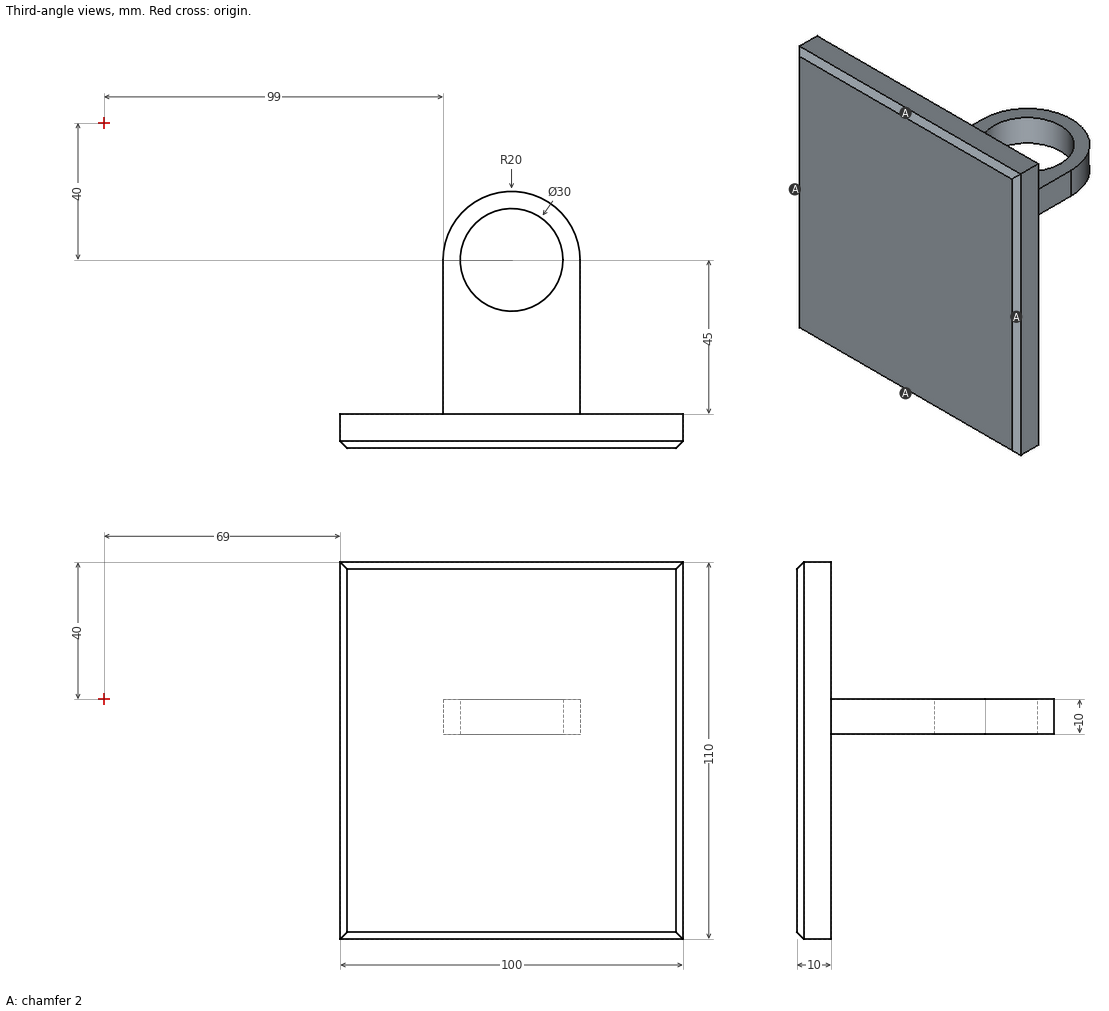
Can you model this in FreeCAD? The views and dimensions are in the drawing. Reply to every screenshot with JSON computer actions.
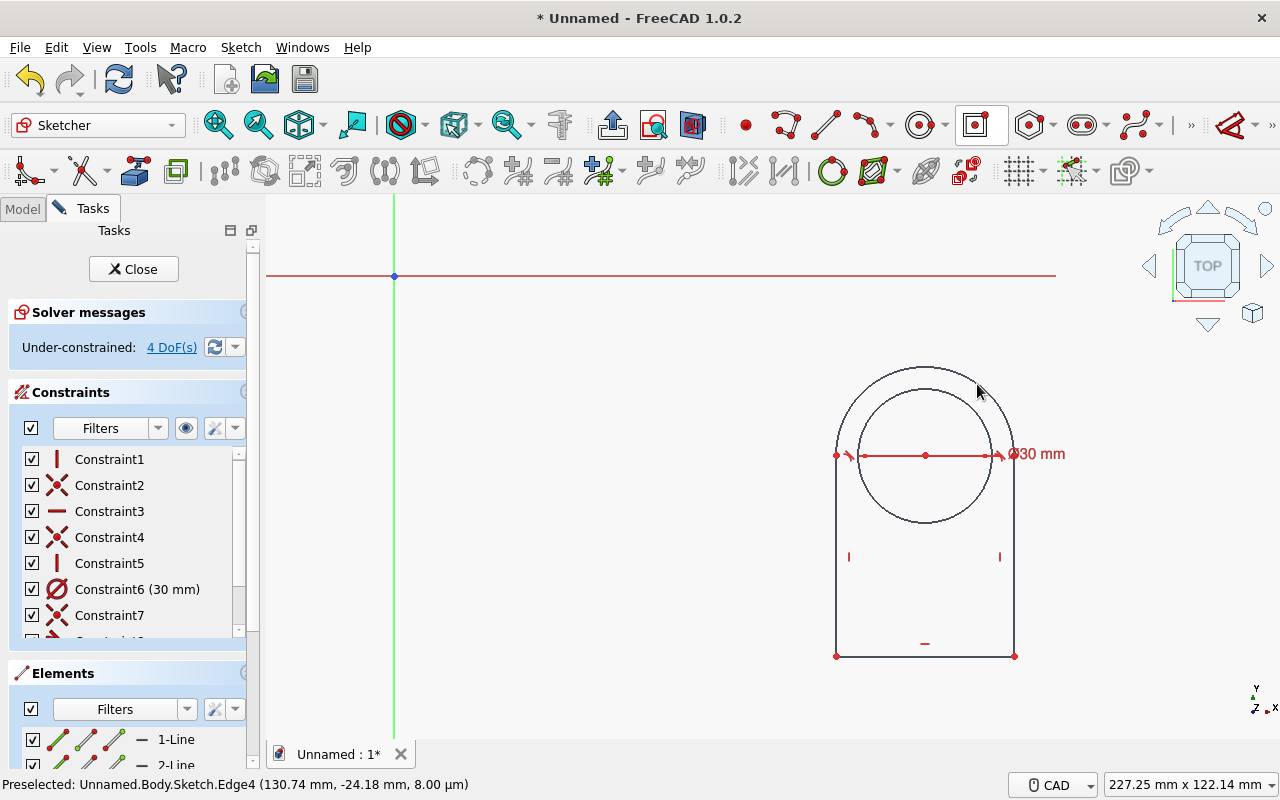
{"action": "left_click", "coordinate": [1230, 126]}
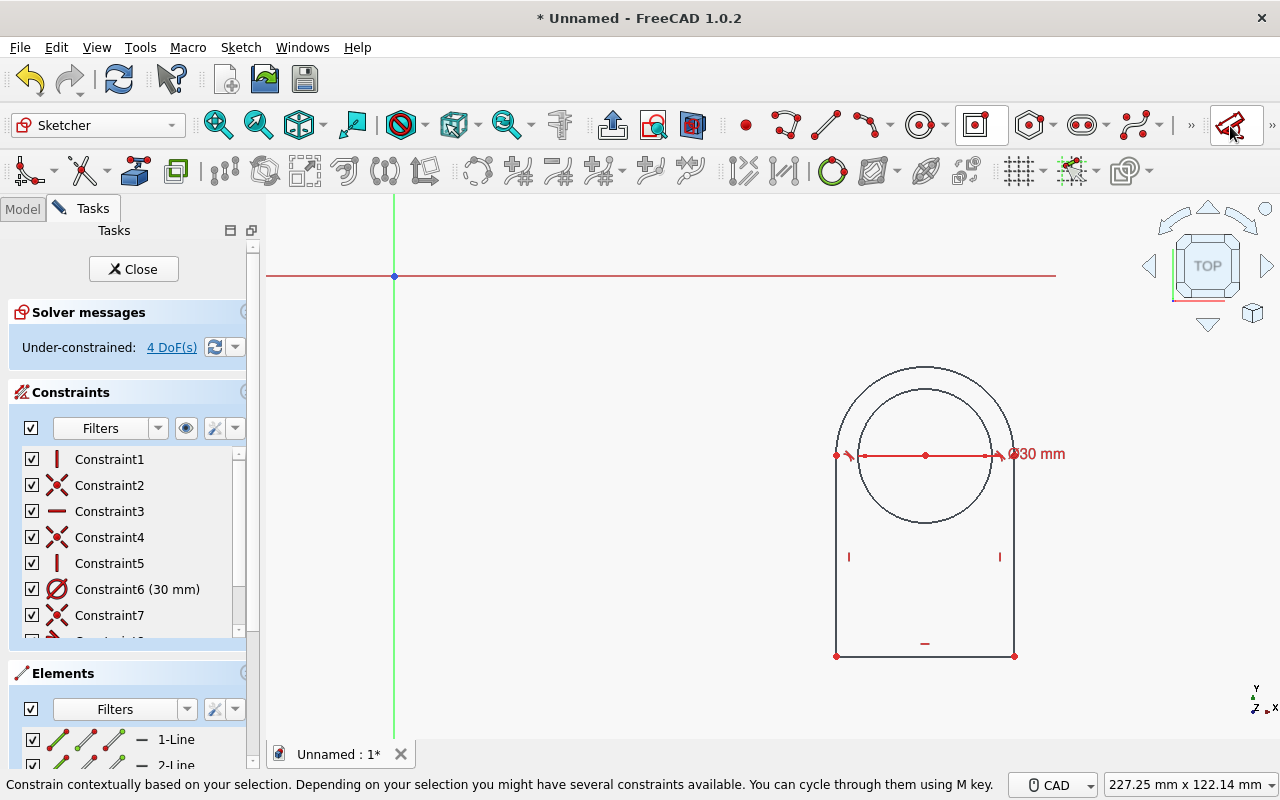
{"action": "left_click", "coordinate": [977, 384]}
{"action": "left_click", "coordinate": [996, 358]}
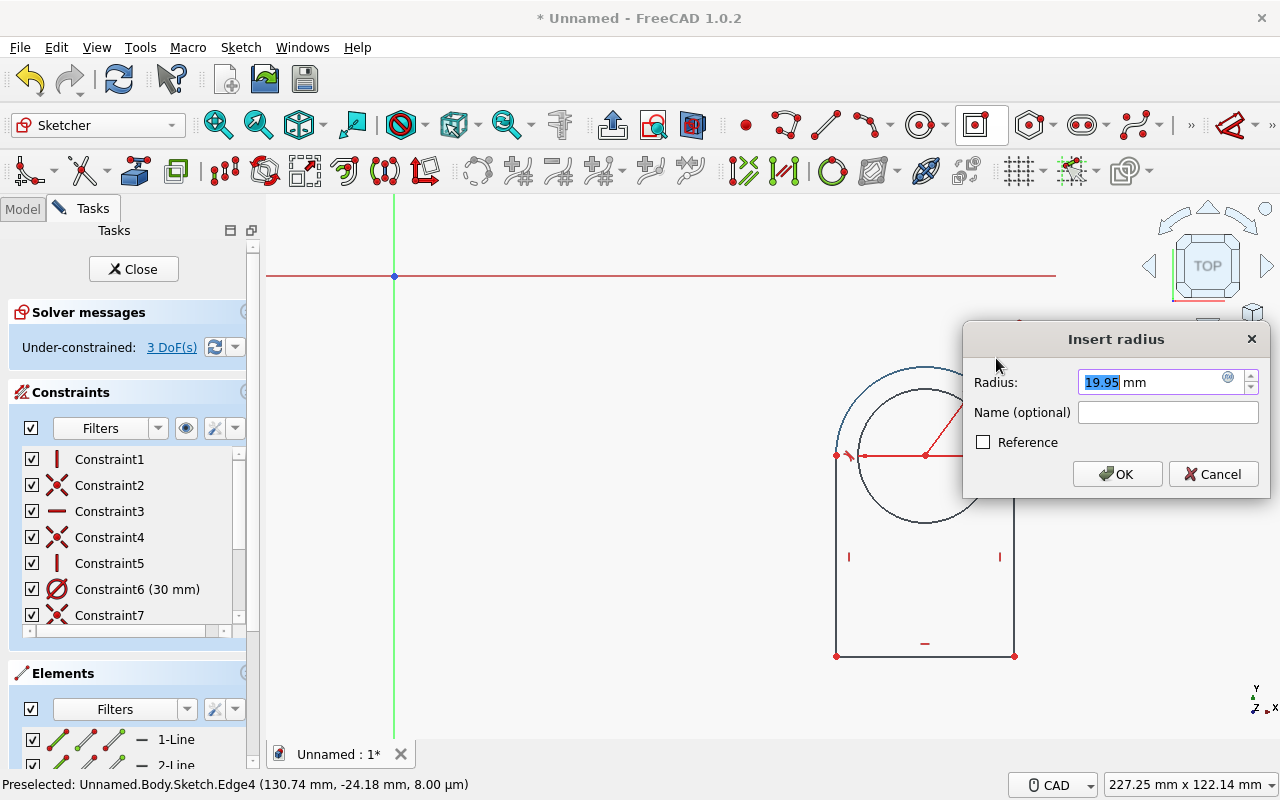
{"action": "type", "text": "20"}
{"action": "key", "text": "Return"}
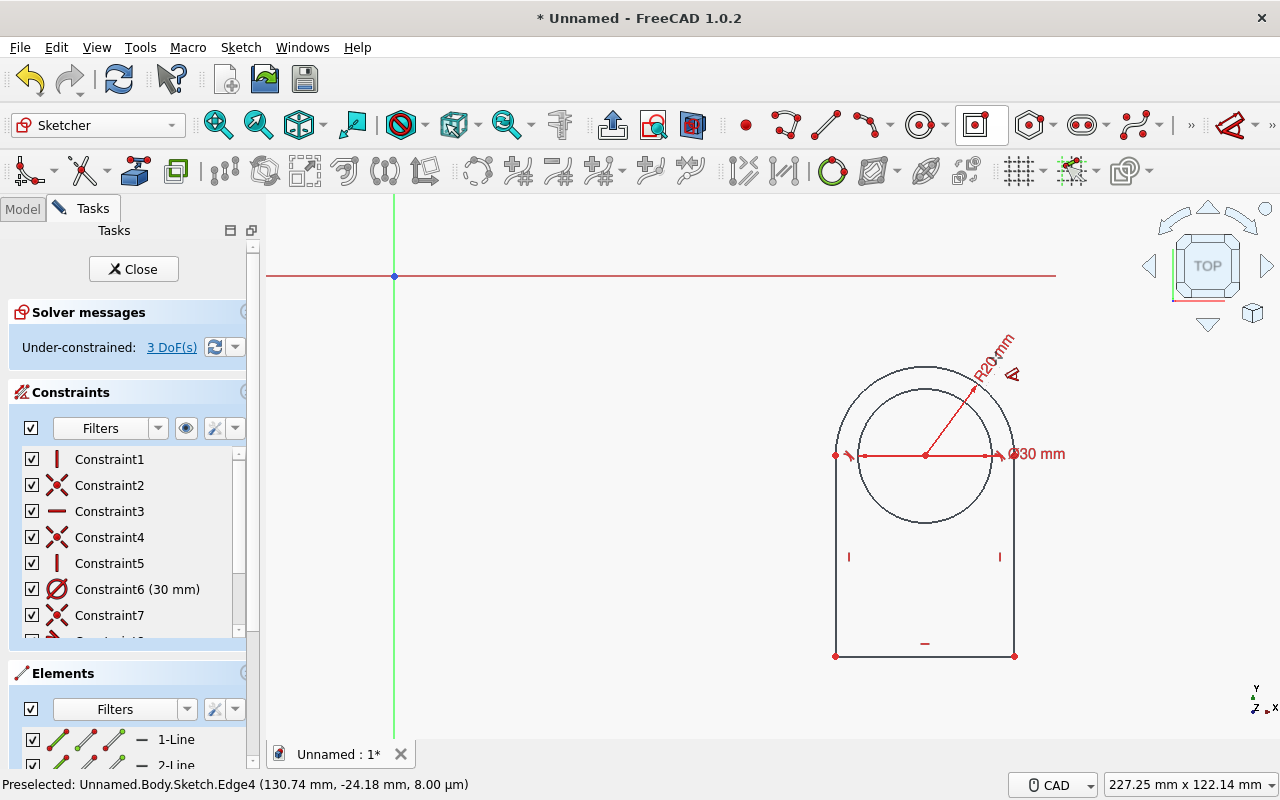
{"action": "left_click", "coordinate": [836, 516]}
{"action": "left_click", "coordinate": [870, 556]}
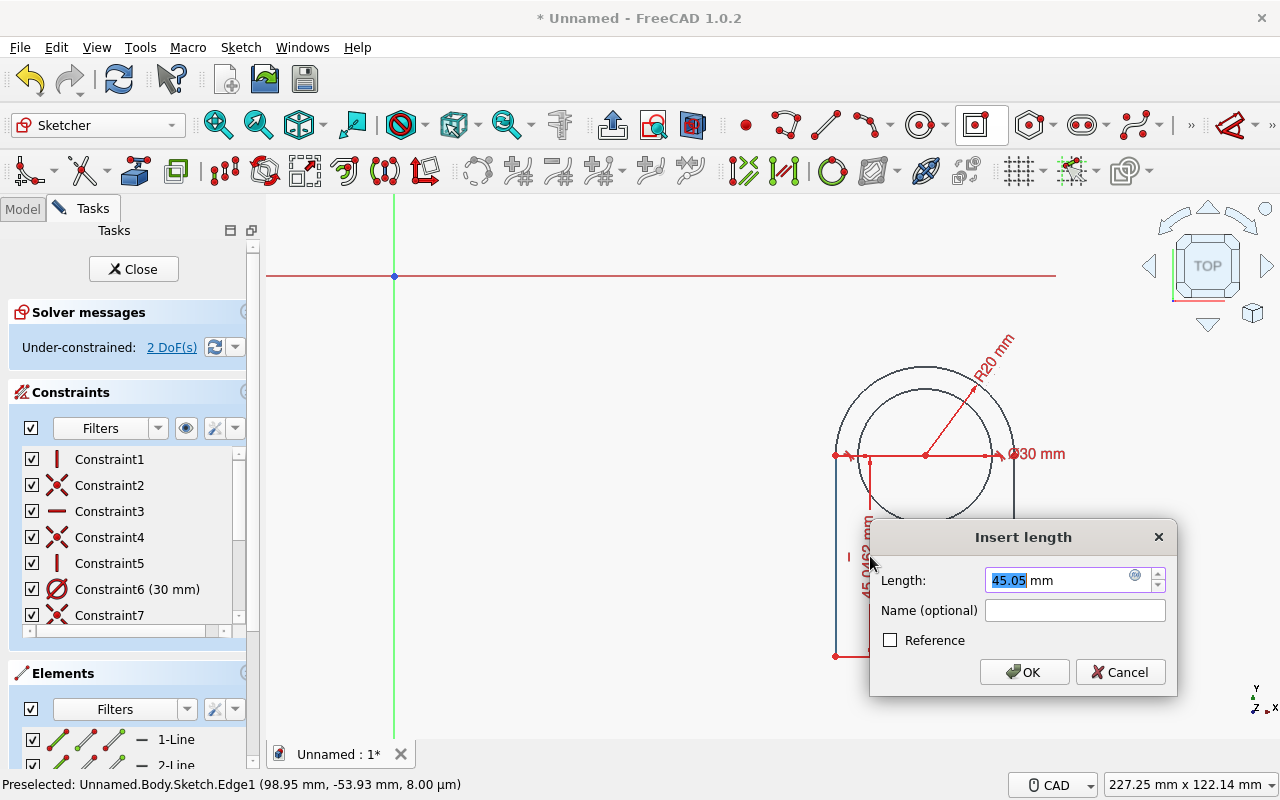
{"action": "type", "text": "45"}
{"action": "key", "text": "Return"}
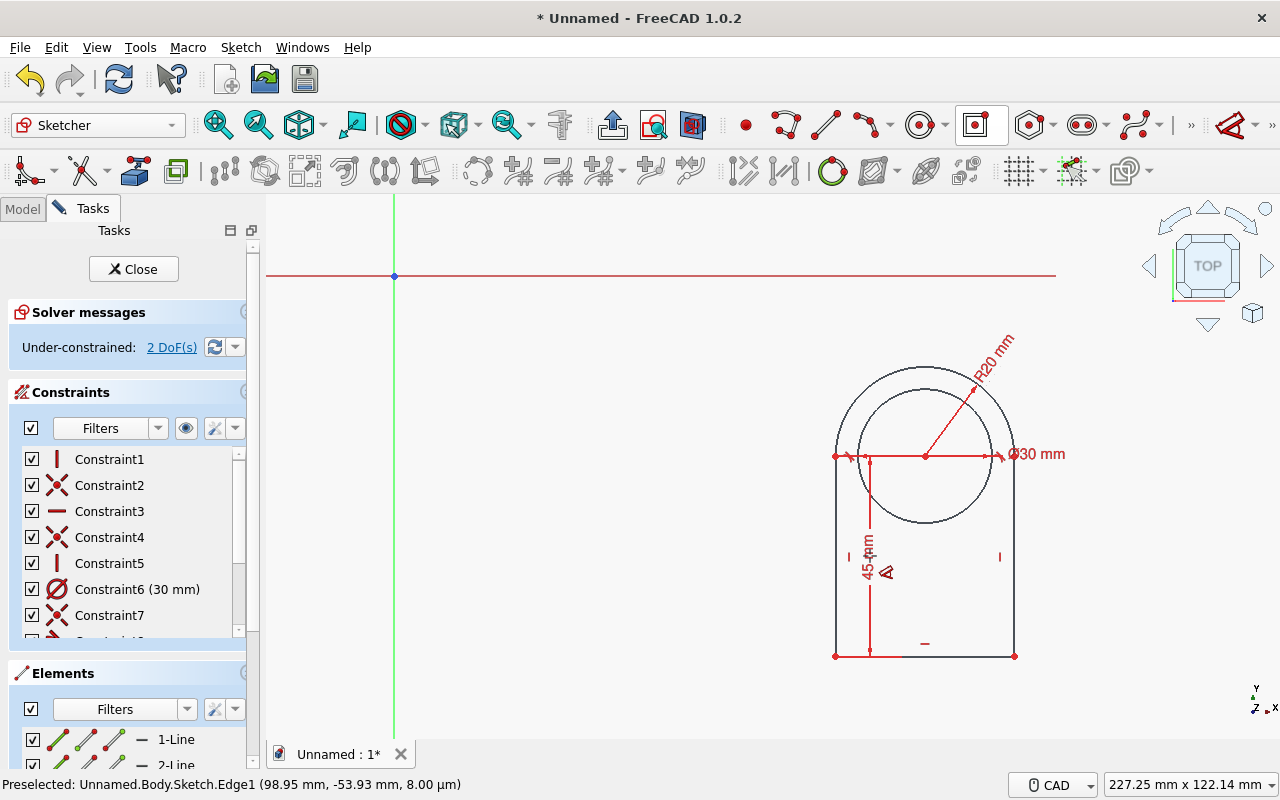
{"action": "left_click", "coordinate": [925, 456]}
{"action": "left_click", "coordinate": [360, 366]}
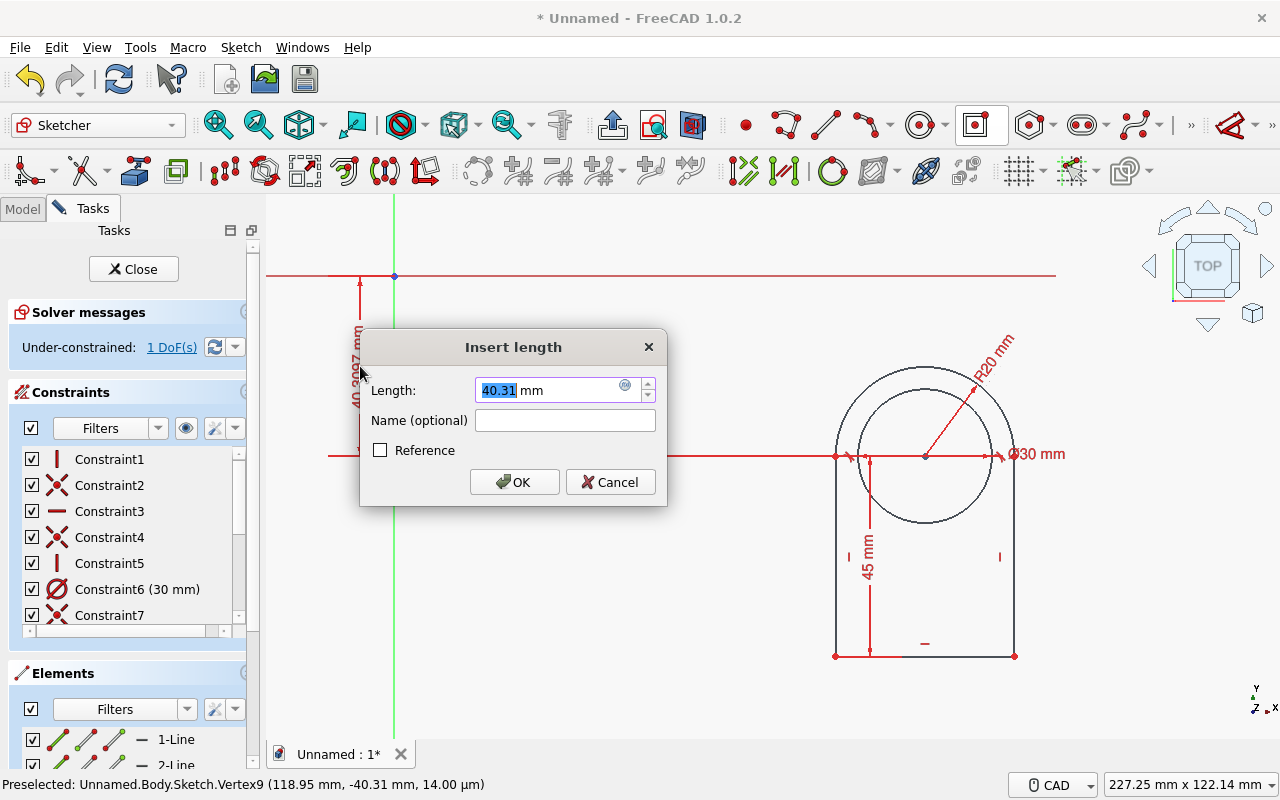
{"action": "type", "text": "40"}
{"action": "key", "text": "Return"}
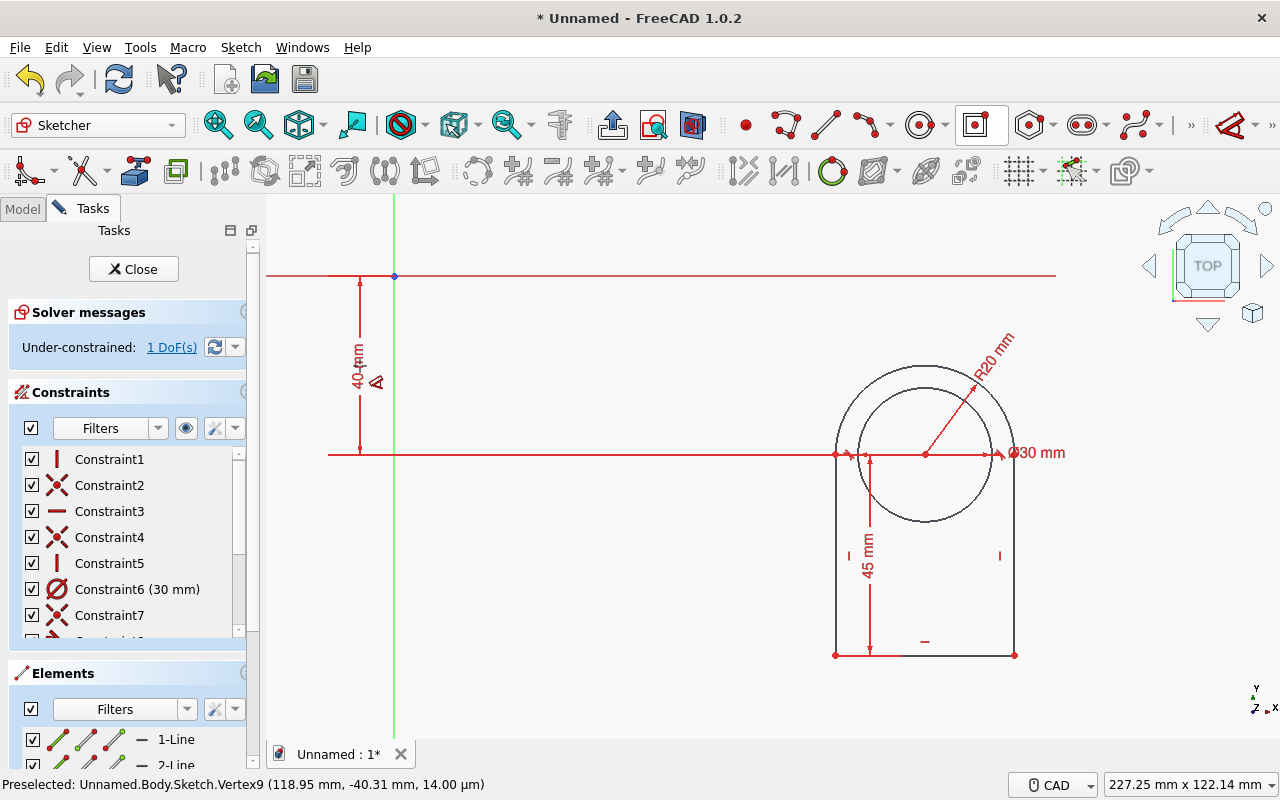
{"action": "left_click", "coordinate": [836, 455]}
{"action": "left_click", "coordinate": [615, 242]}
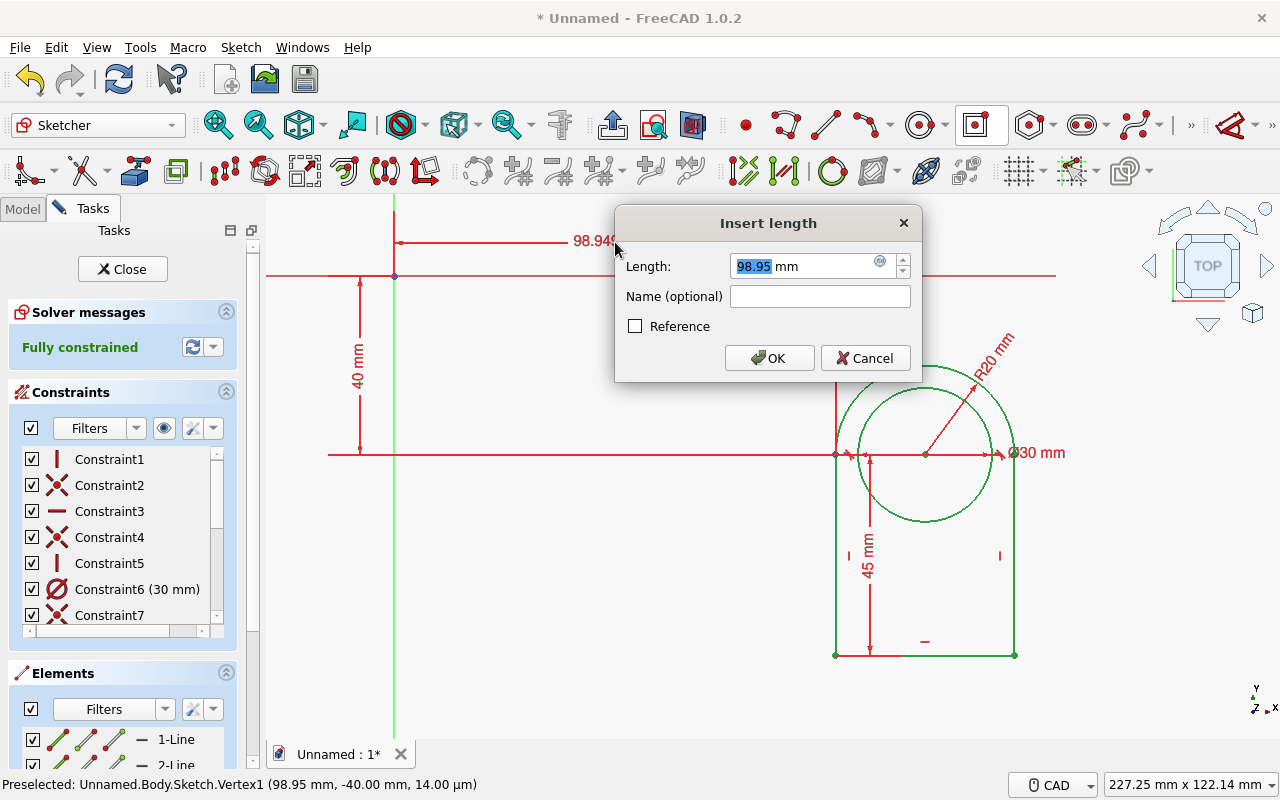
{"action": "type", "text": "99"}
{"action": "key", "text": "Return"}
{"action": "key", "text": "Escape"}